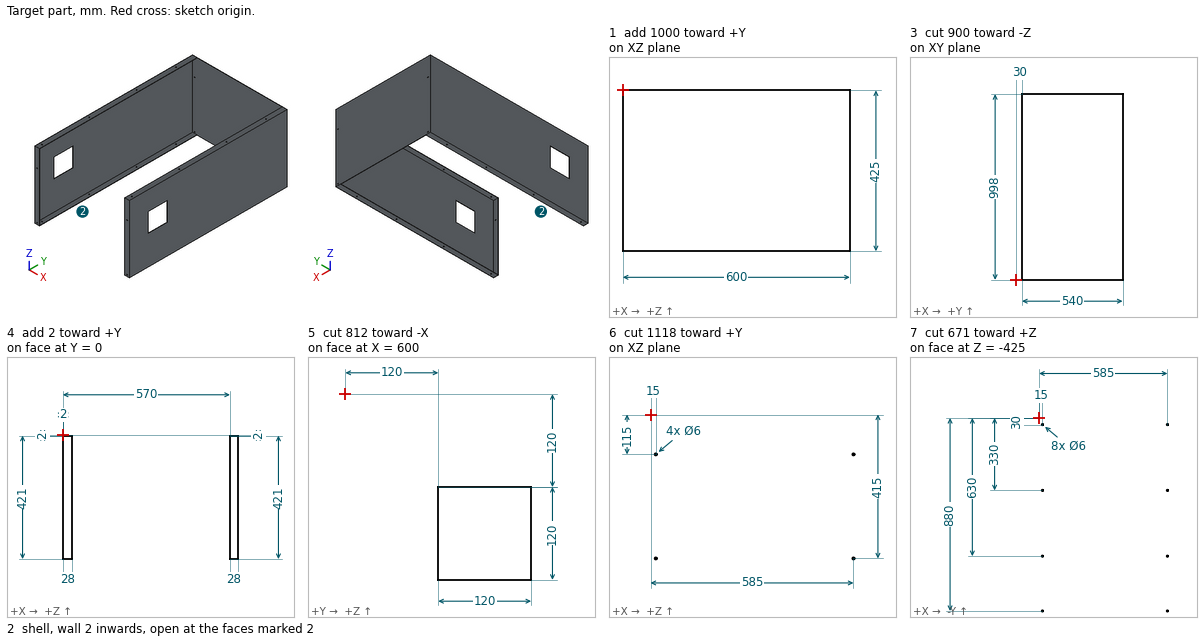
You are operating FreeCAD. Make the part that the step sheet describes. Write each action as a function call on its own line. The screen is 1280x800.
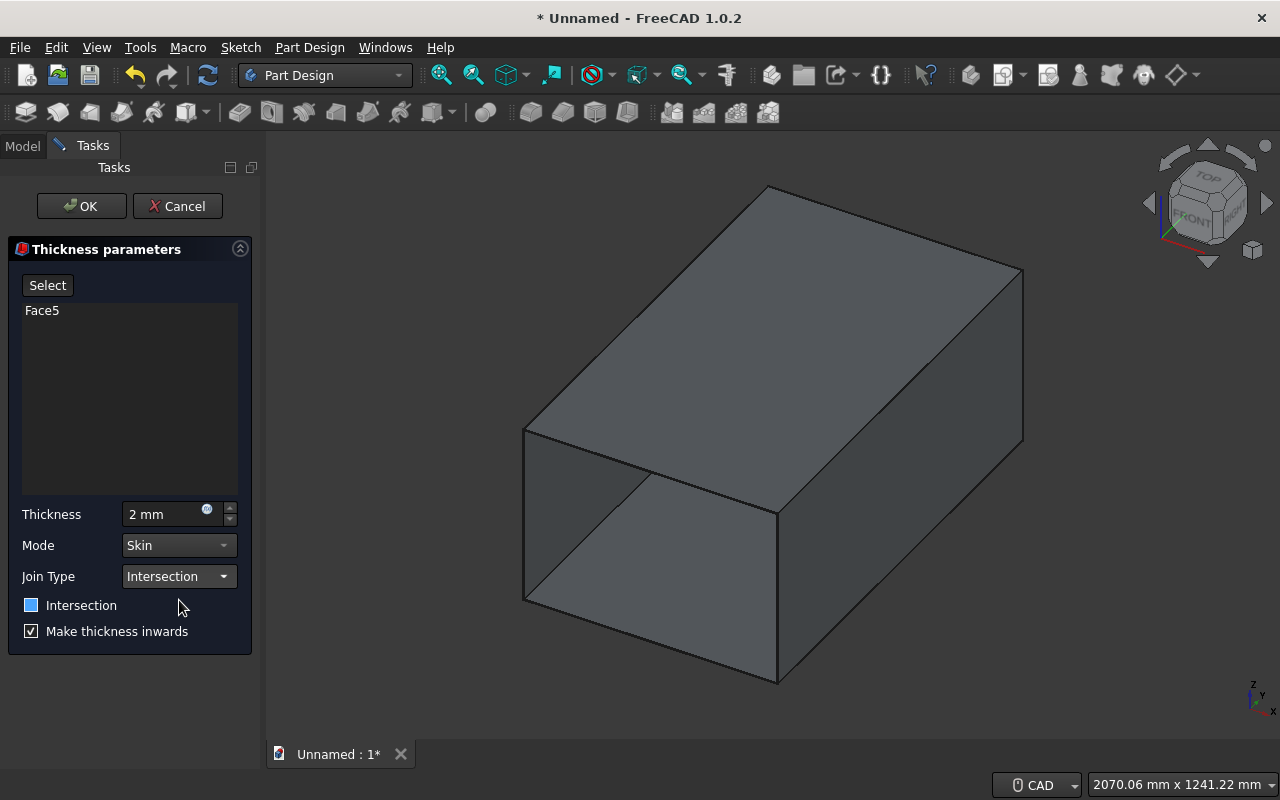
click(82, 206)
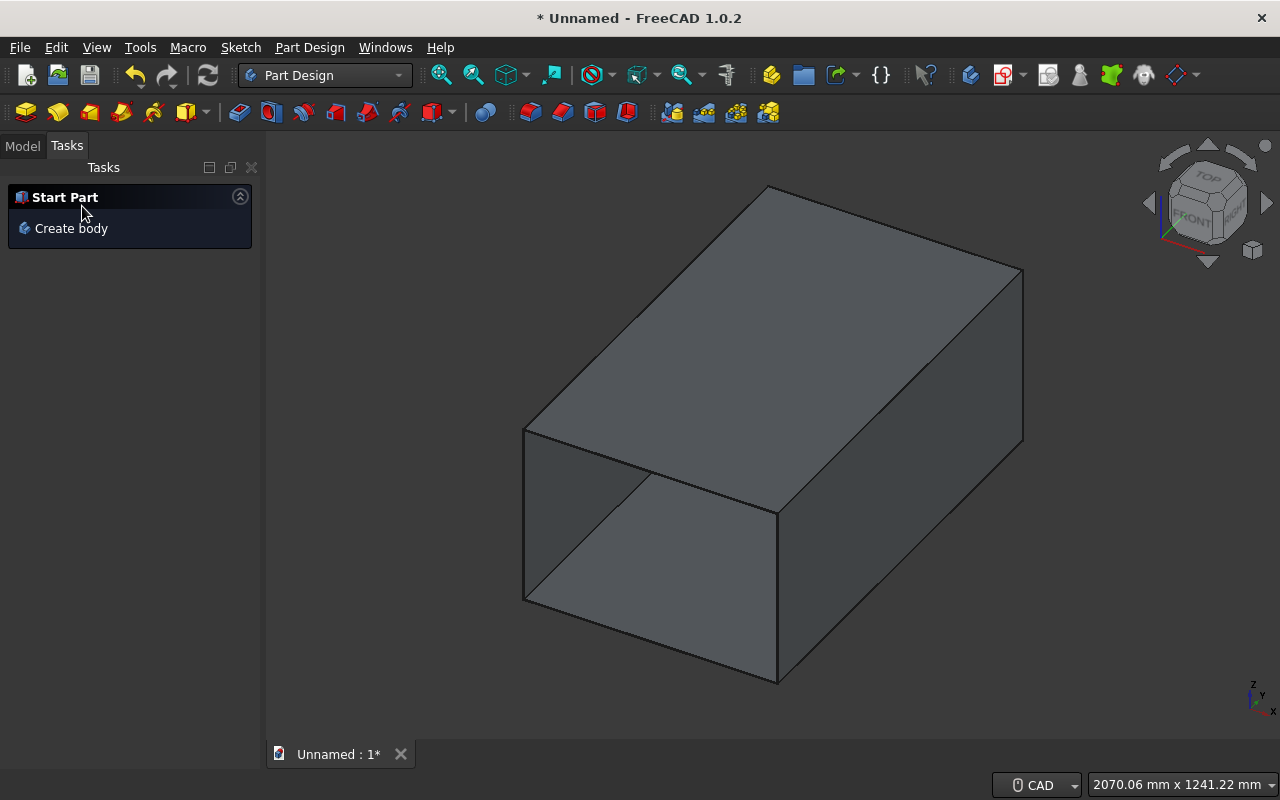
click(1004, 76)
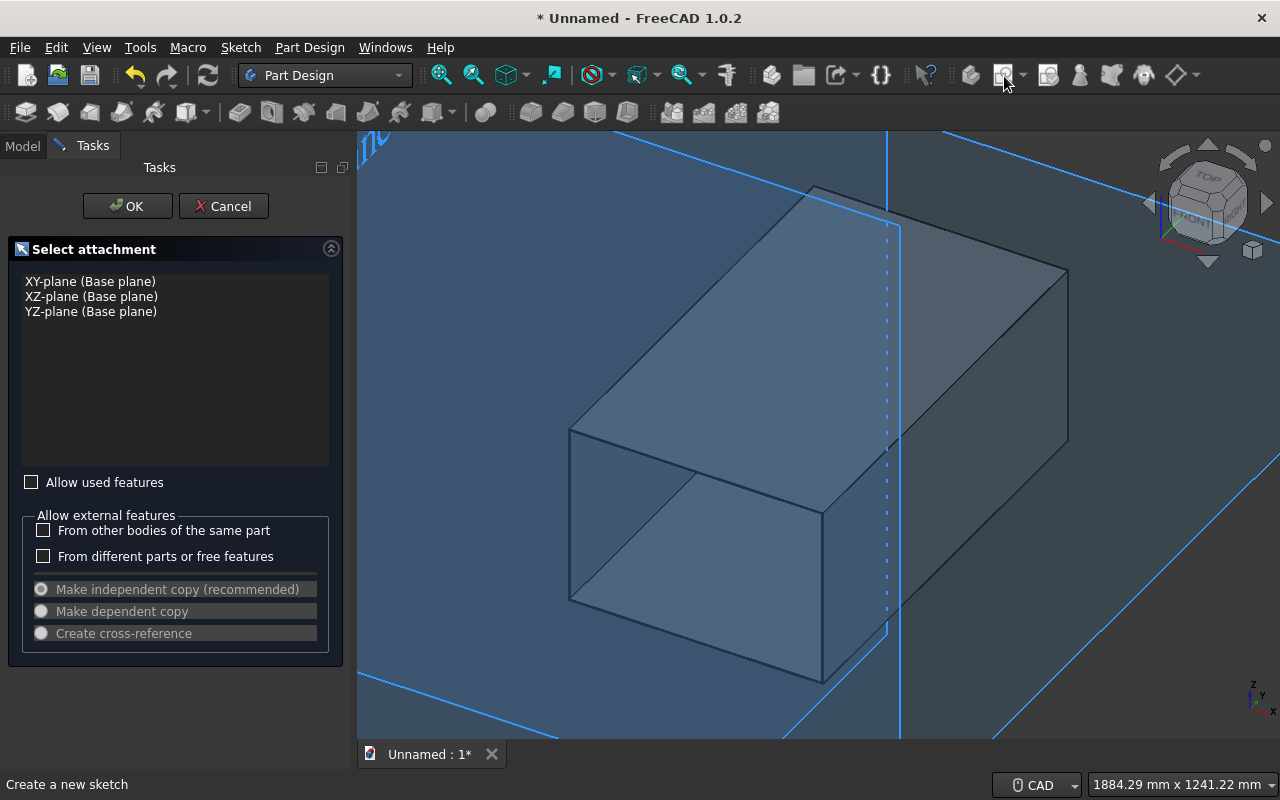
click(82, 282)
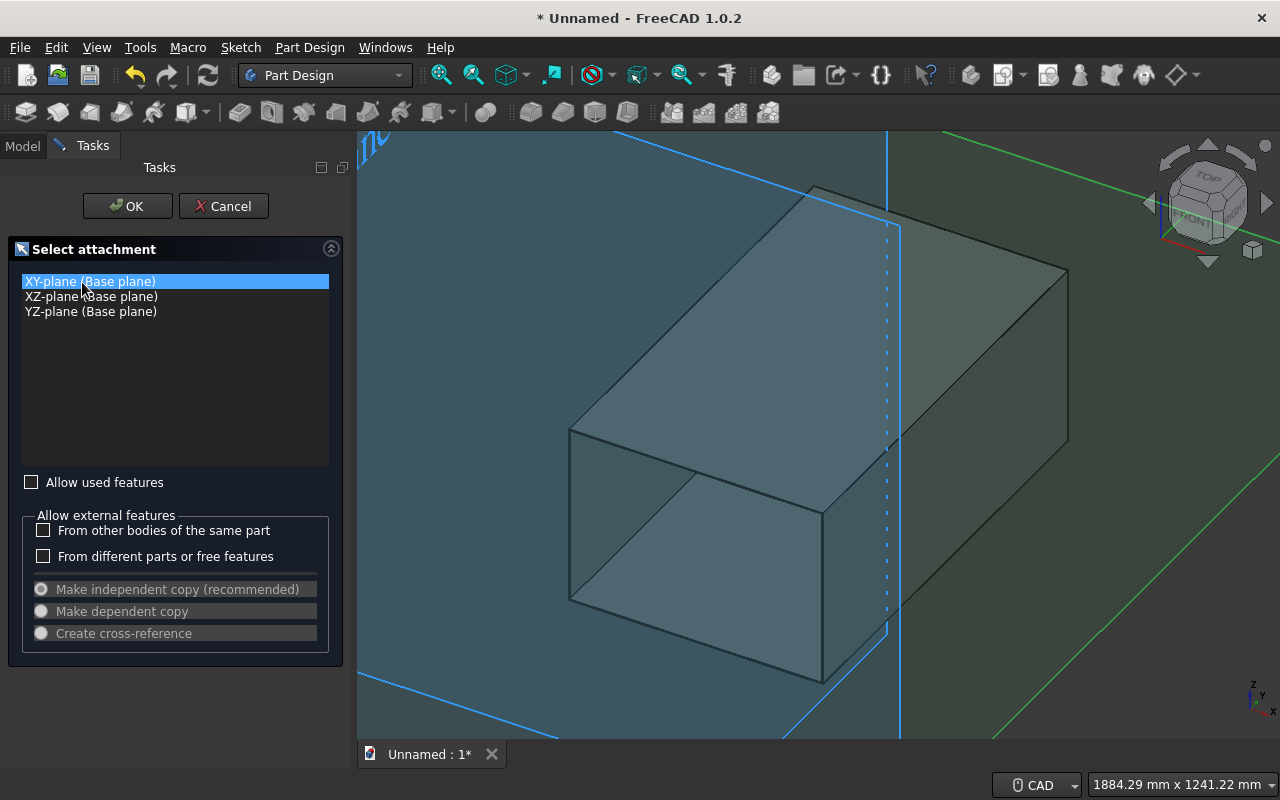
click(128, 206)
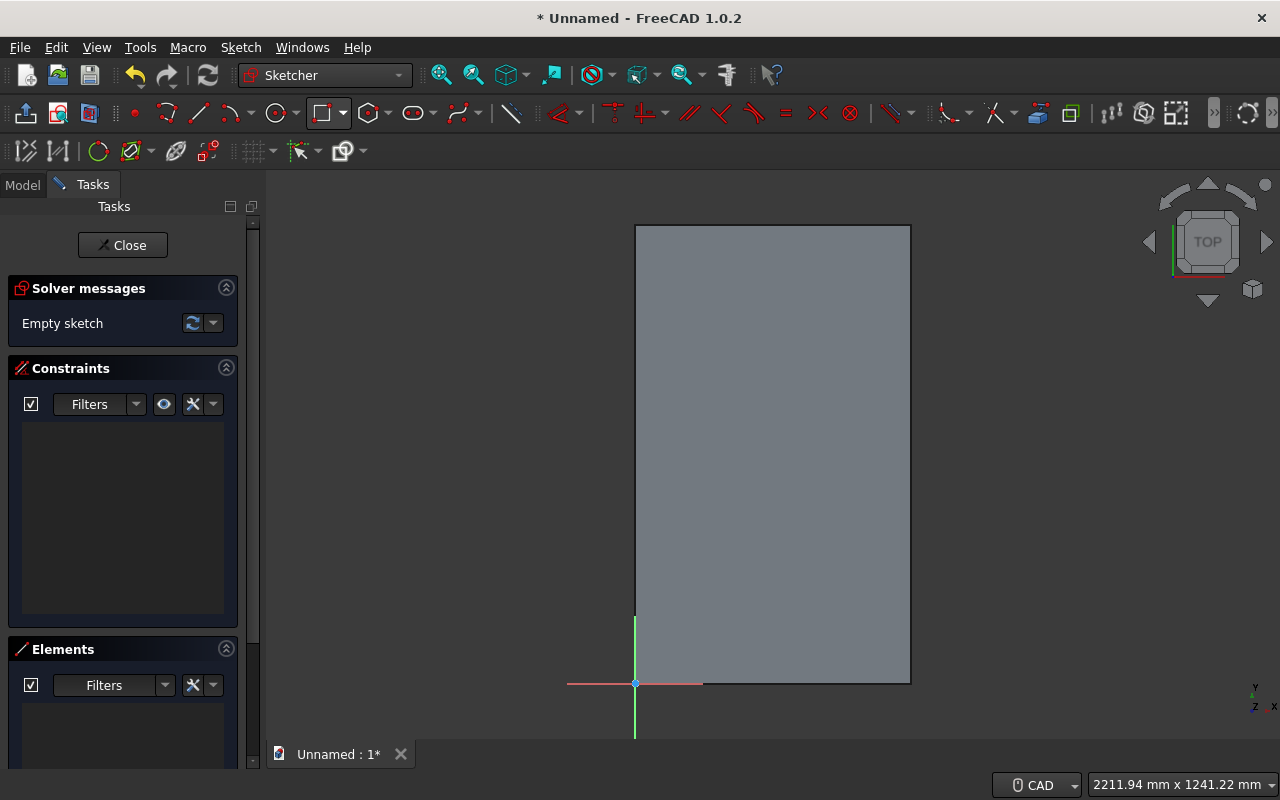
click(322, 114)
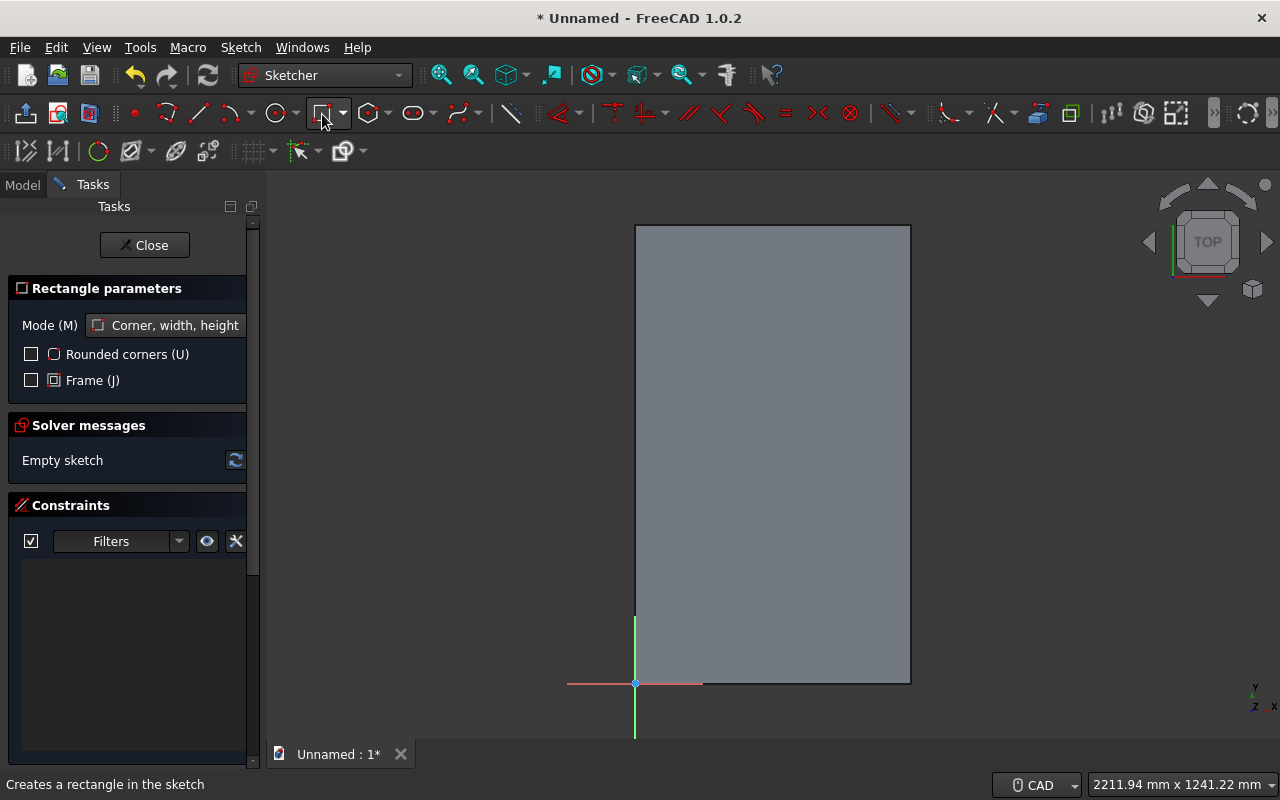
click(649, 226)
click(897, 684)
key(Escape)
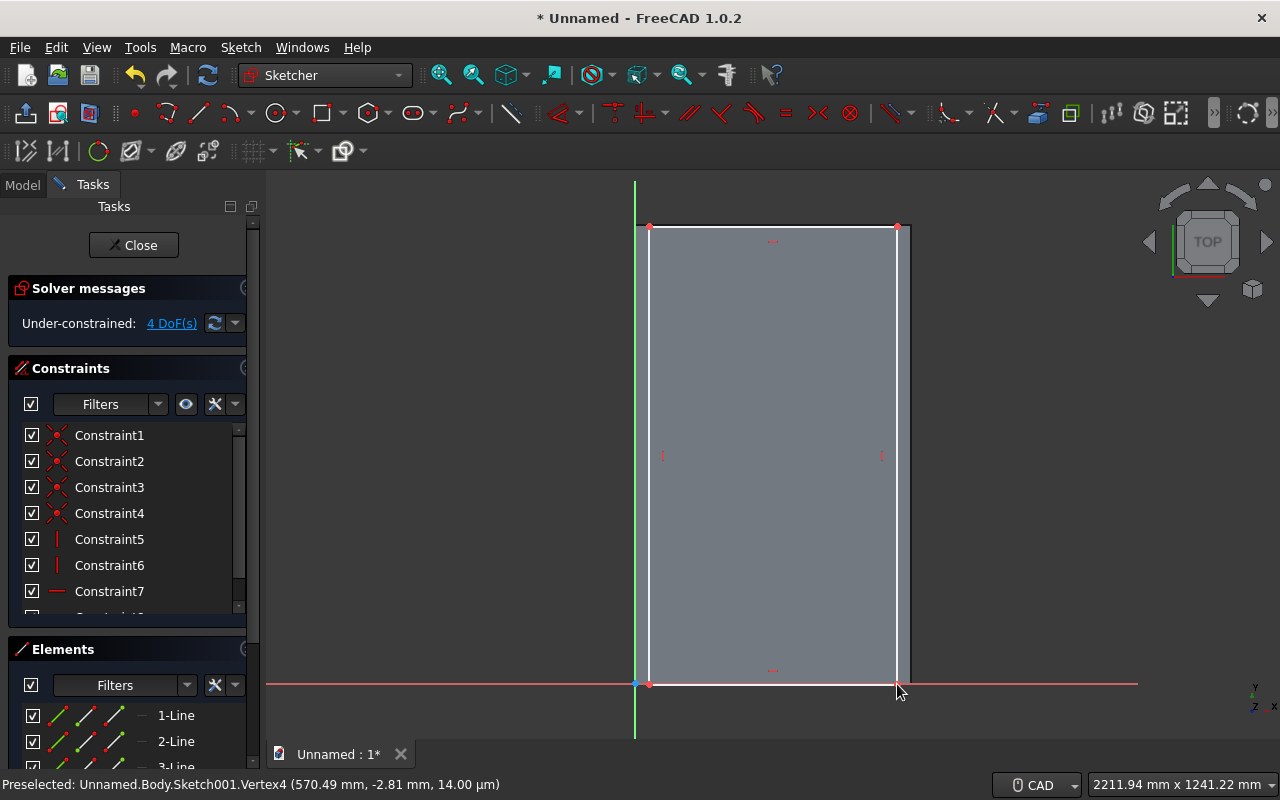
click(649, 685)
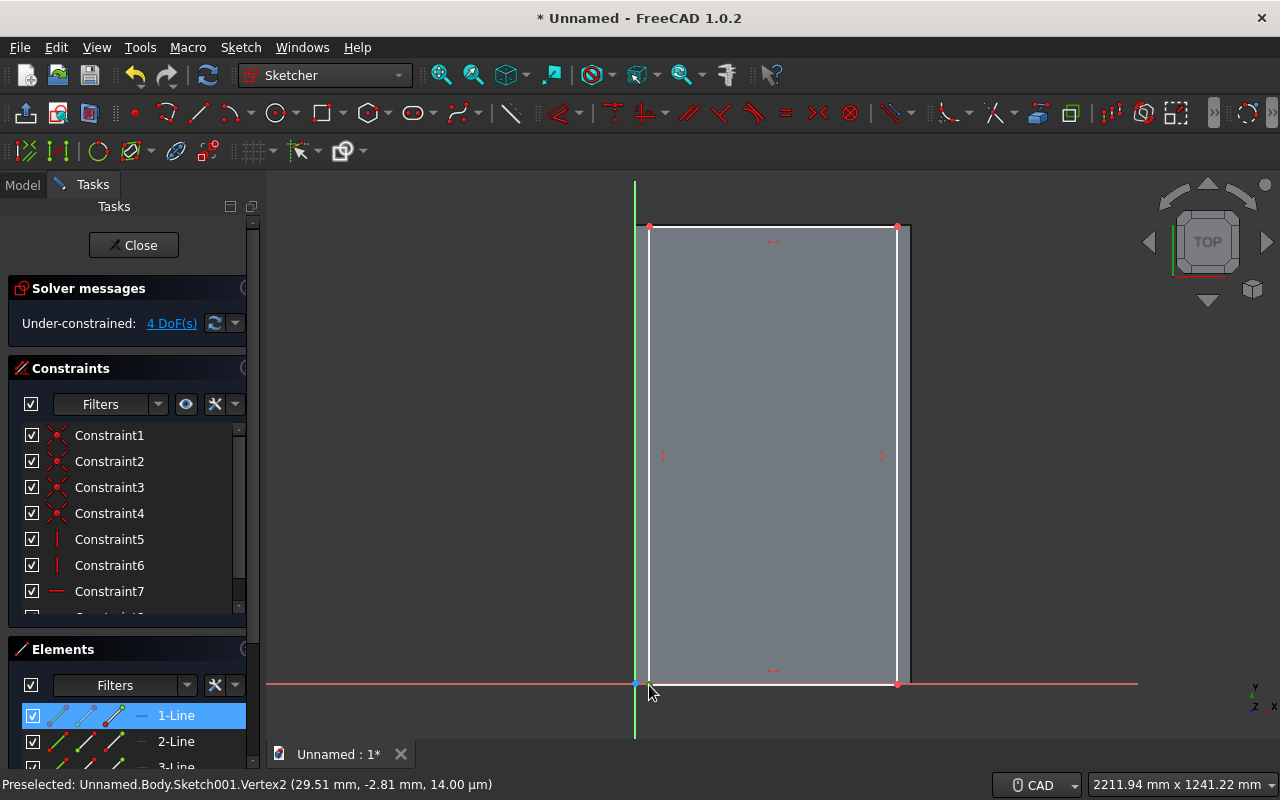
click(353, 684)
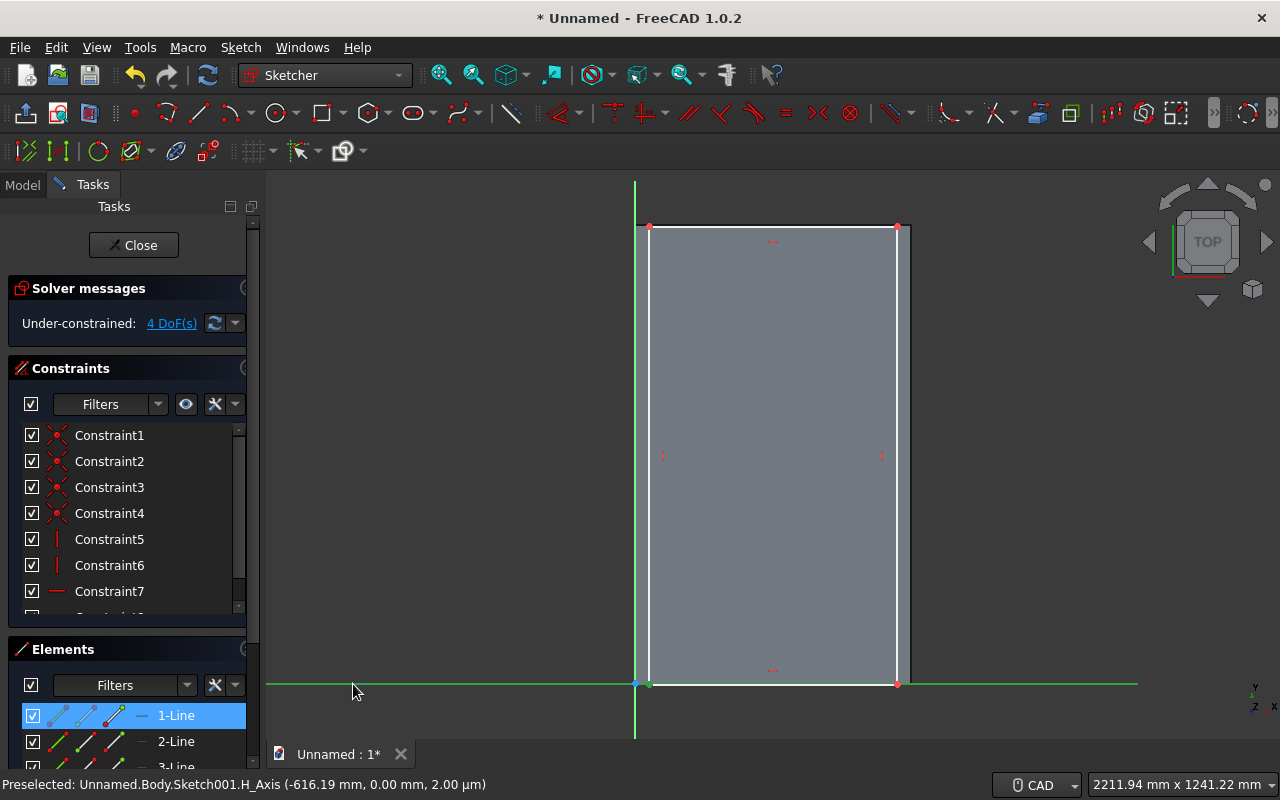
click(614, 114)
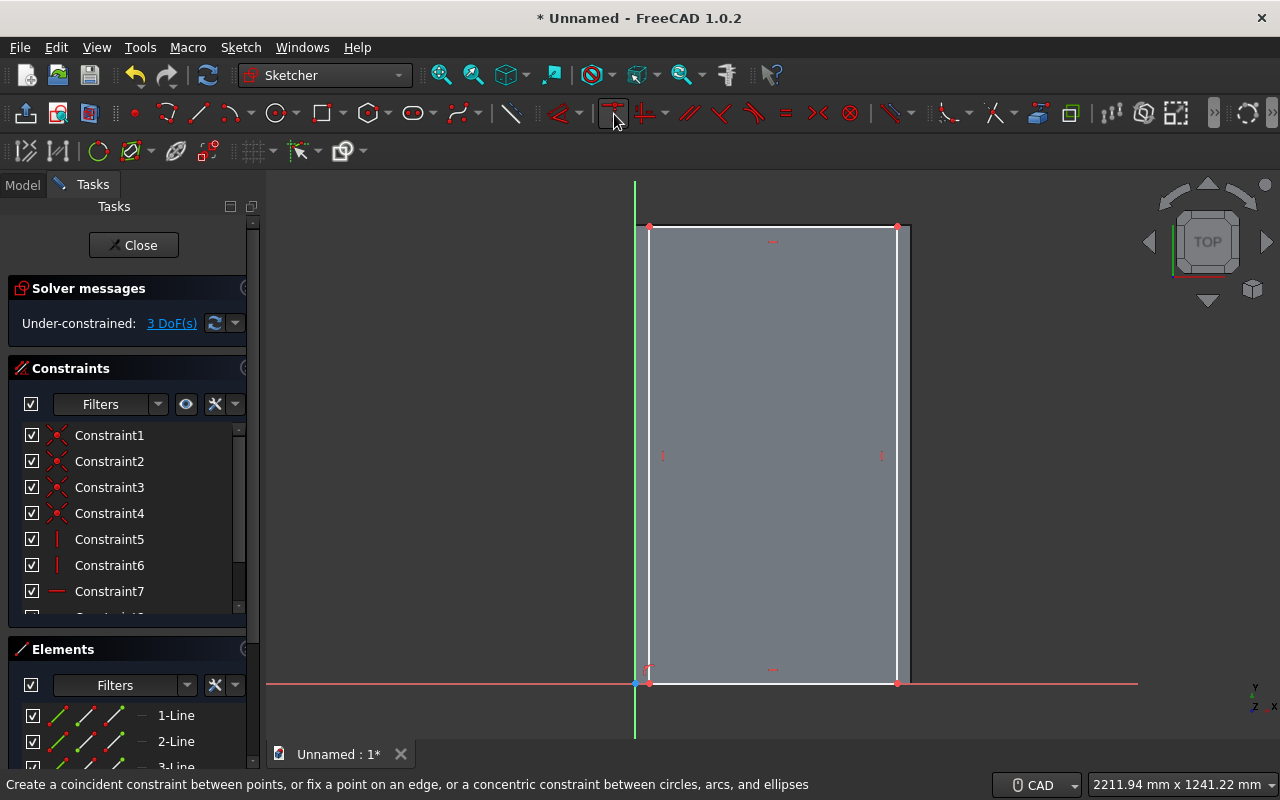
click(558, 114)